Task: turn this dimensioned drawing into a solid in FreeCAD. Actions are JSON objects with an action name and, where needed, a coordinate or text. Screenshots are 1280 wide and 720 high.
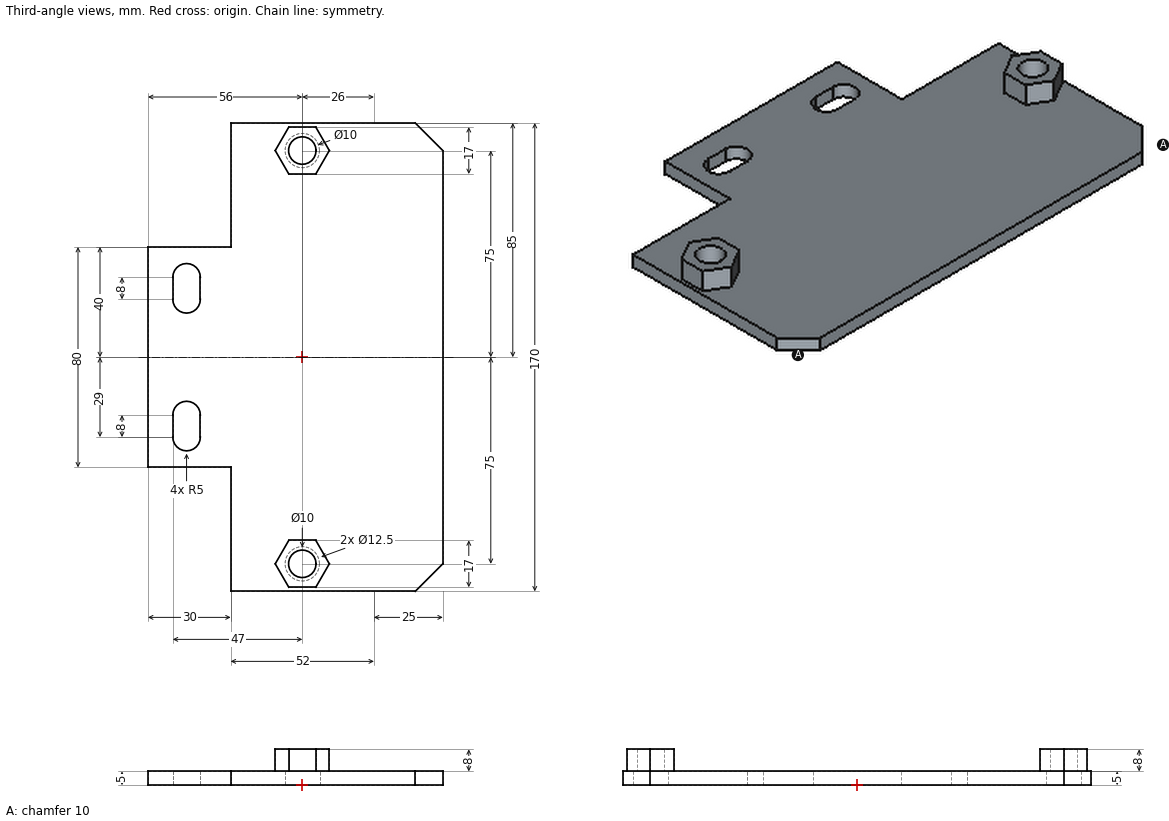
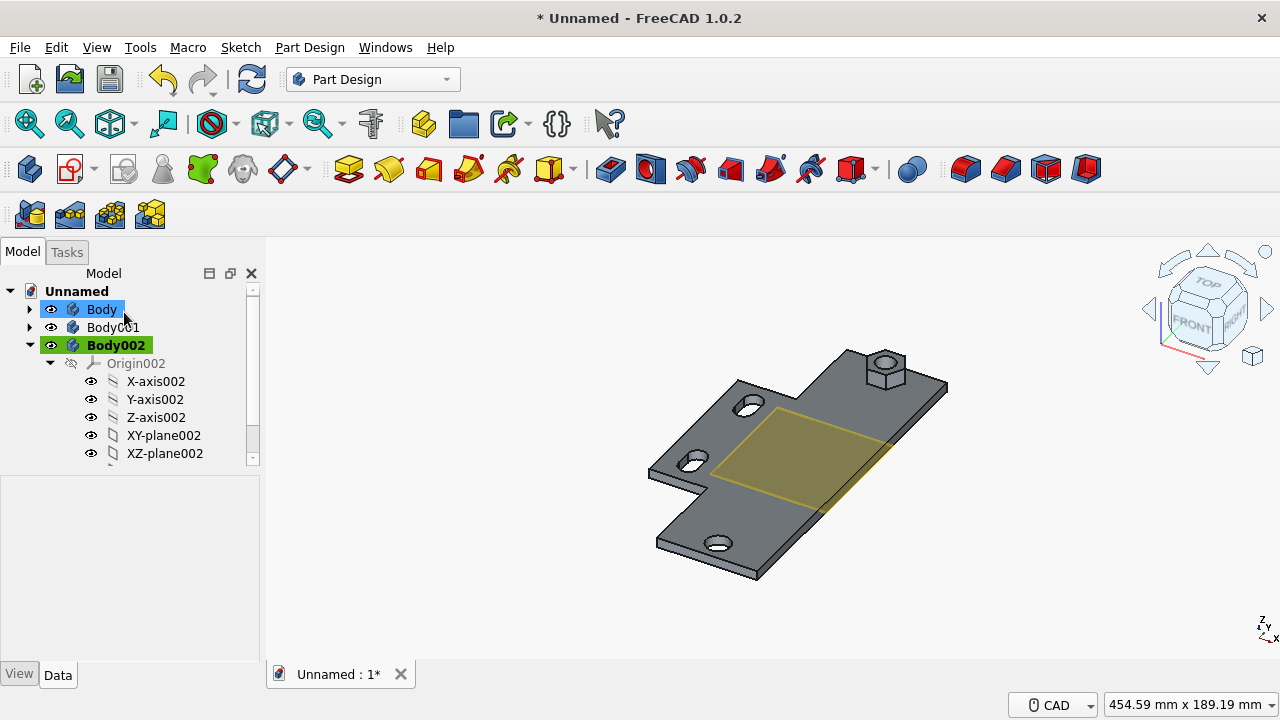
{"action": "scroll", "coordinate": [100, 377], "scroll_direction": "down", "scroll_amount": 3}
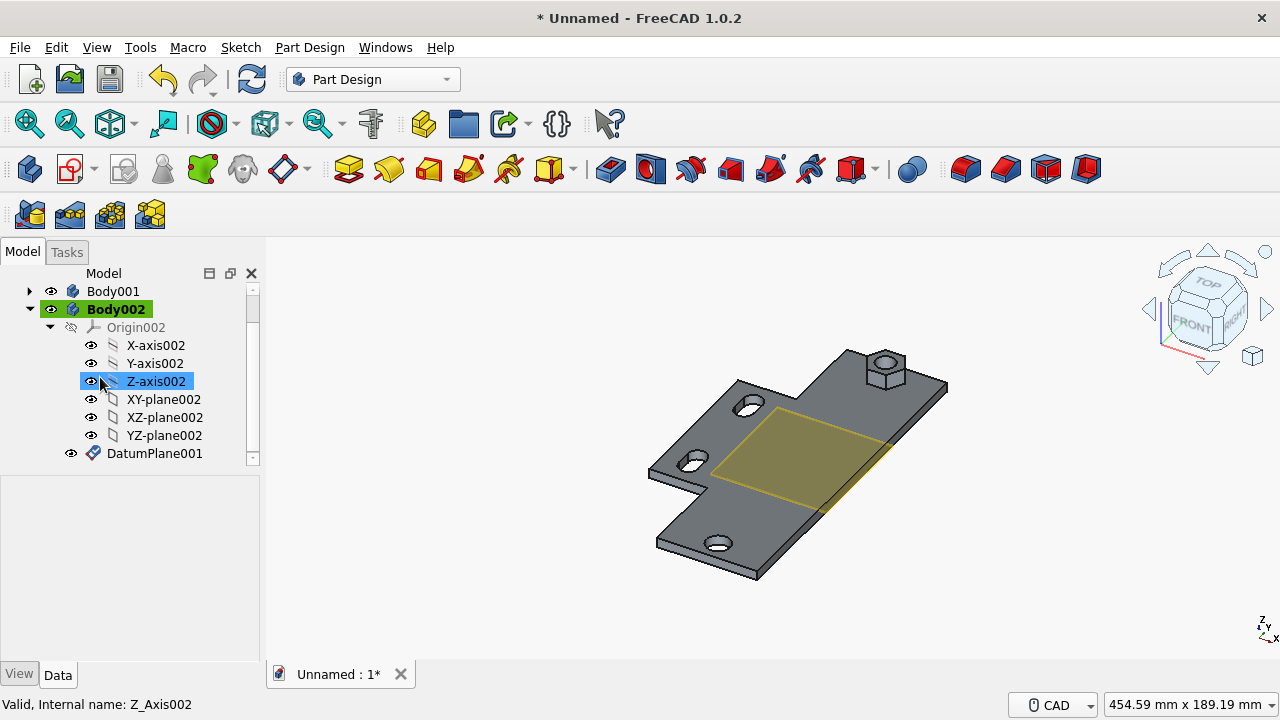
{"action": "left_click", "coordinate": [116, 453]}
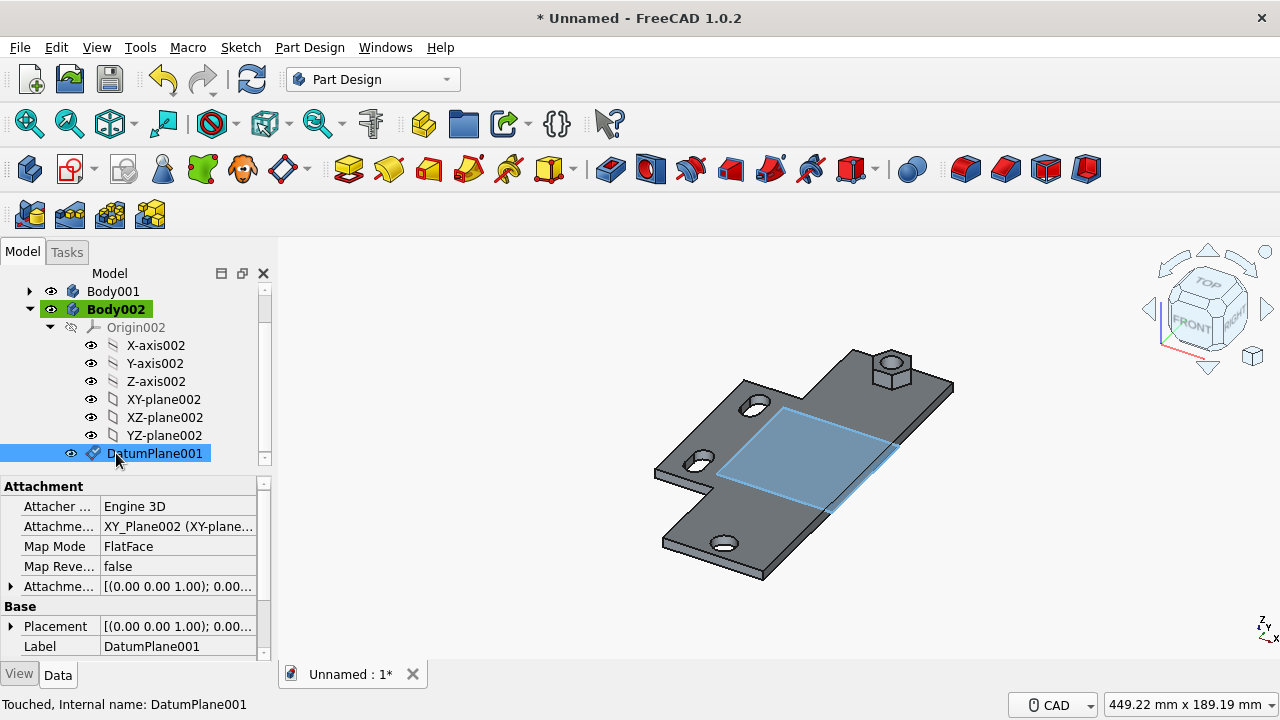
{"action": "left_click", "coordinate": [70, 170]}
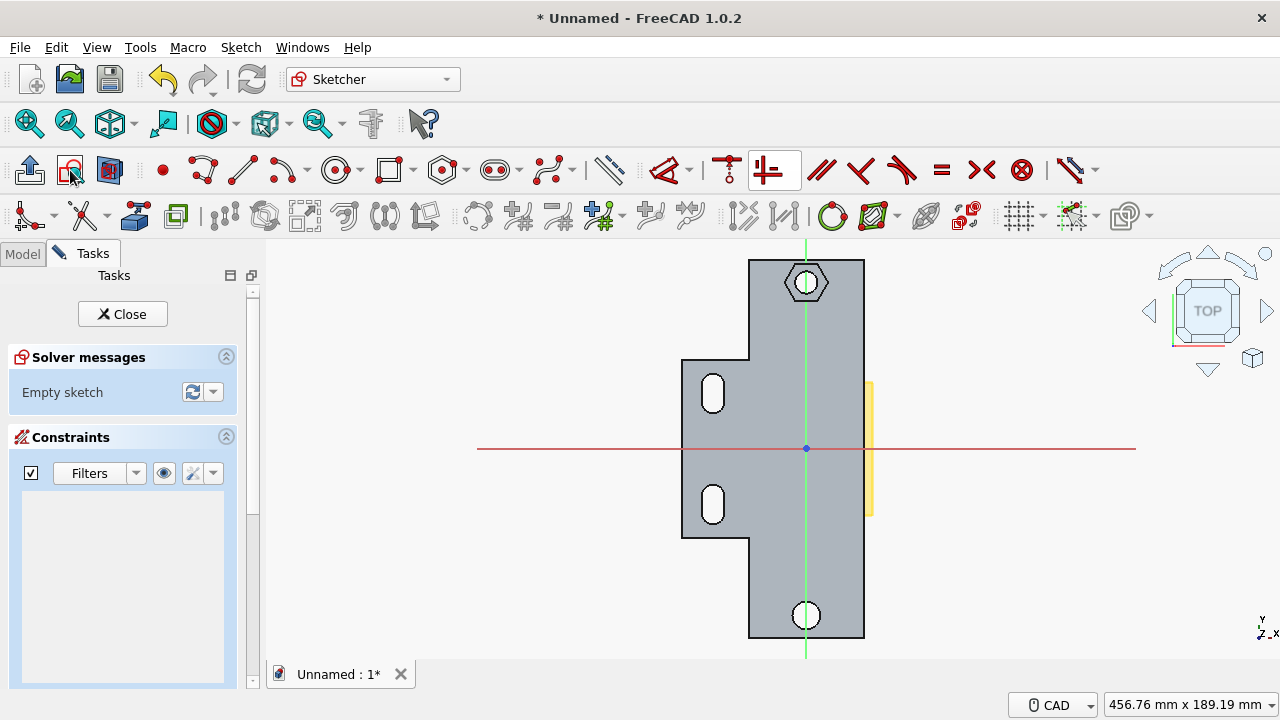
{"action": "scroll", "coordinate": [704, 449], "scroll_direction": "down", "scroll_amount": 5}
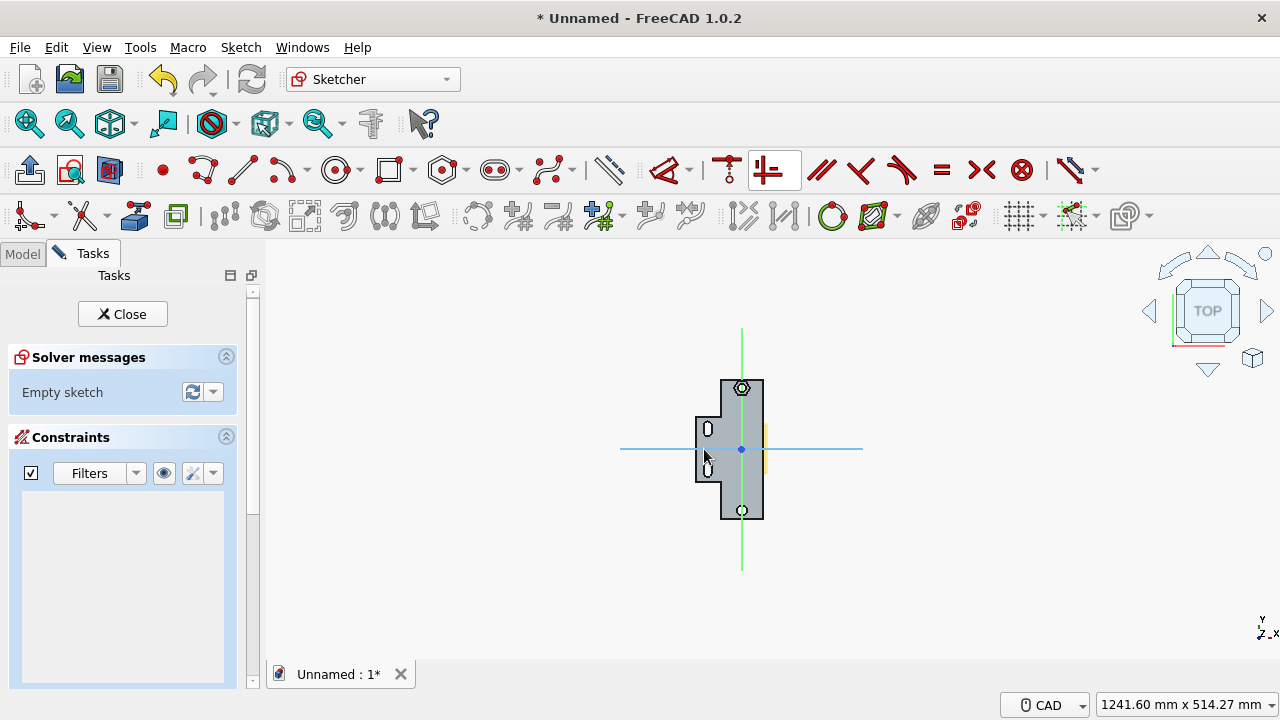
{"action": "scroll", "coordinate": [744, 514], "scroll_direction": "up", "scroll_amount": 15}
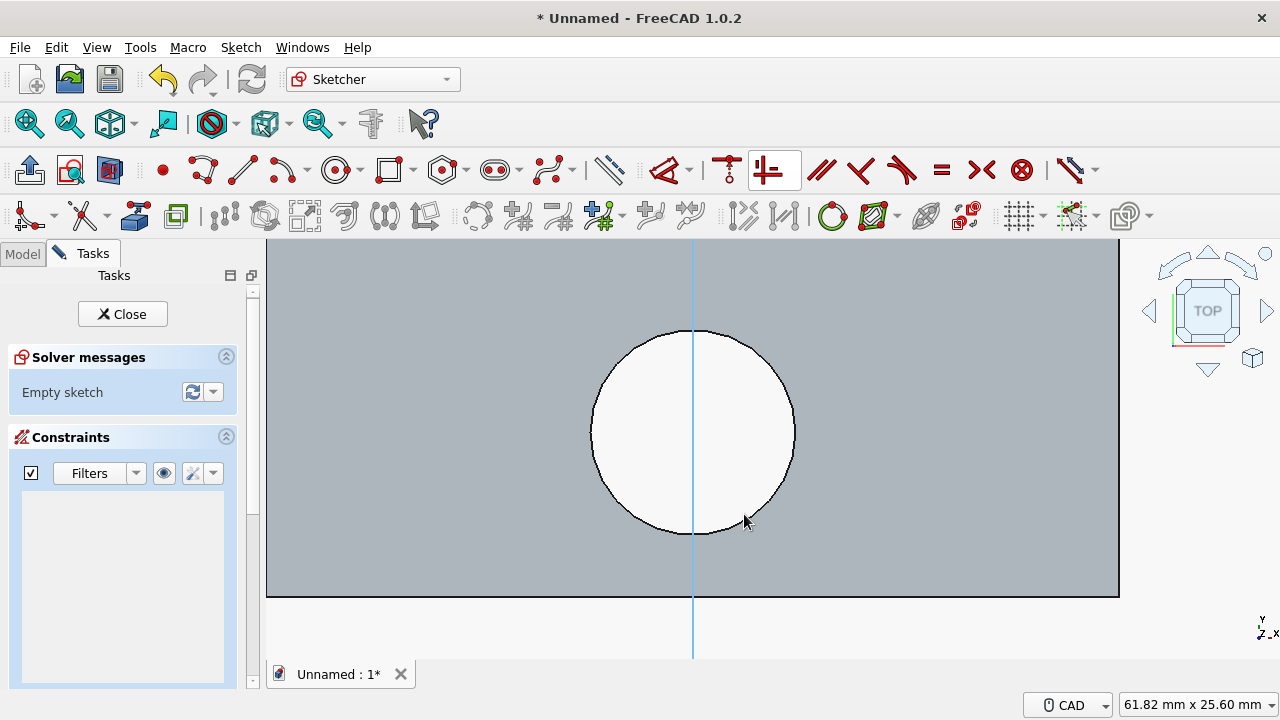
{"action": "left_click", "coordinate": [442, 170]}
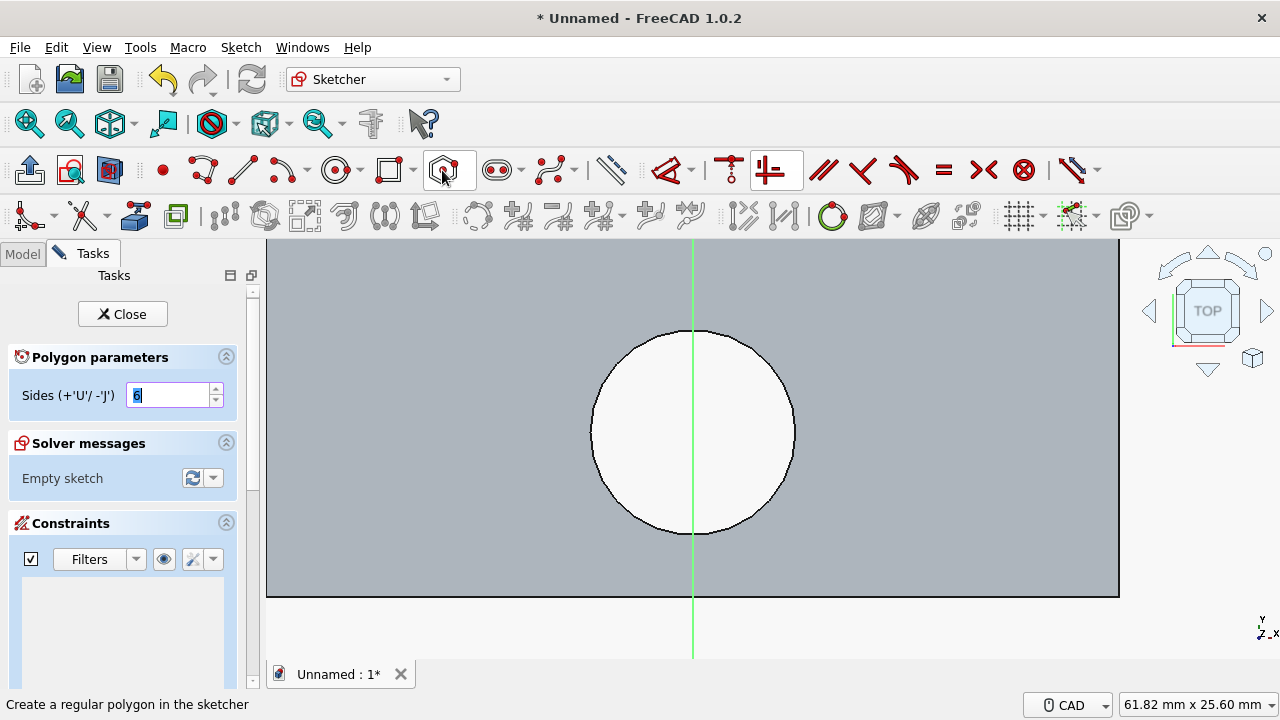
{"action": "left_click", "coordinate": [693, 433]}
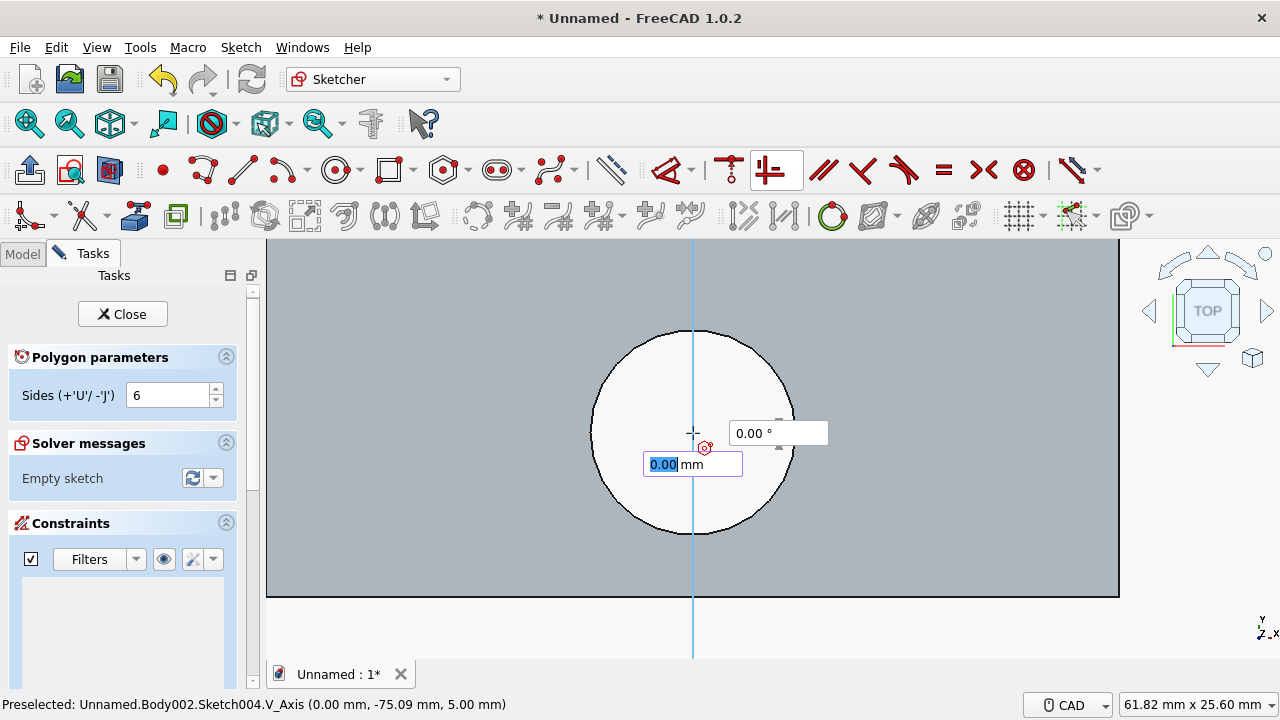
{"action": "left_click", "coordinate": [854, 433]}
{"action": "key", "text": "Escape"}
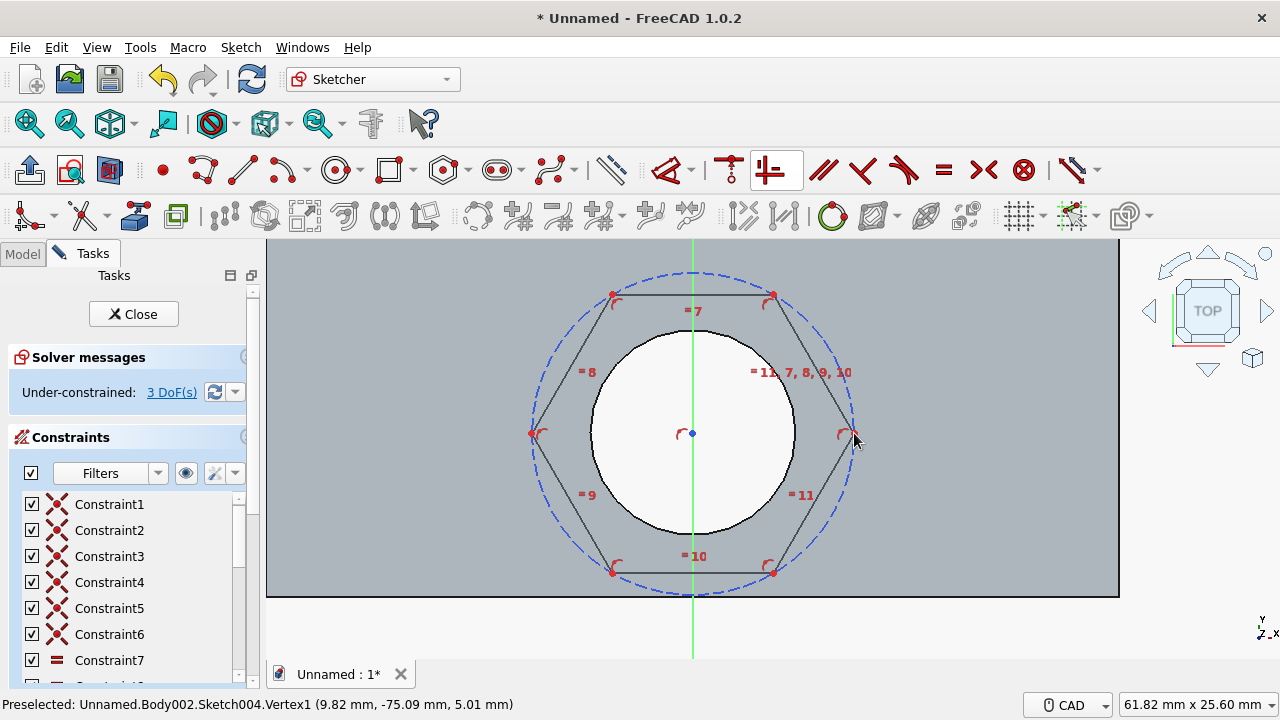
{"action": "left_click", "coordinate": [336, 170]}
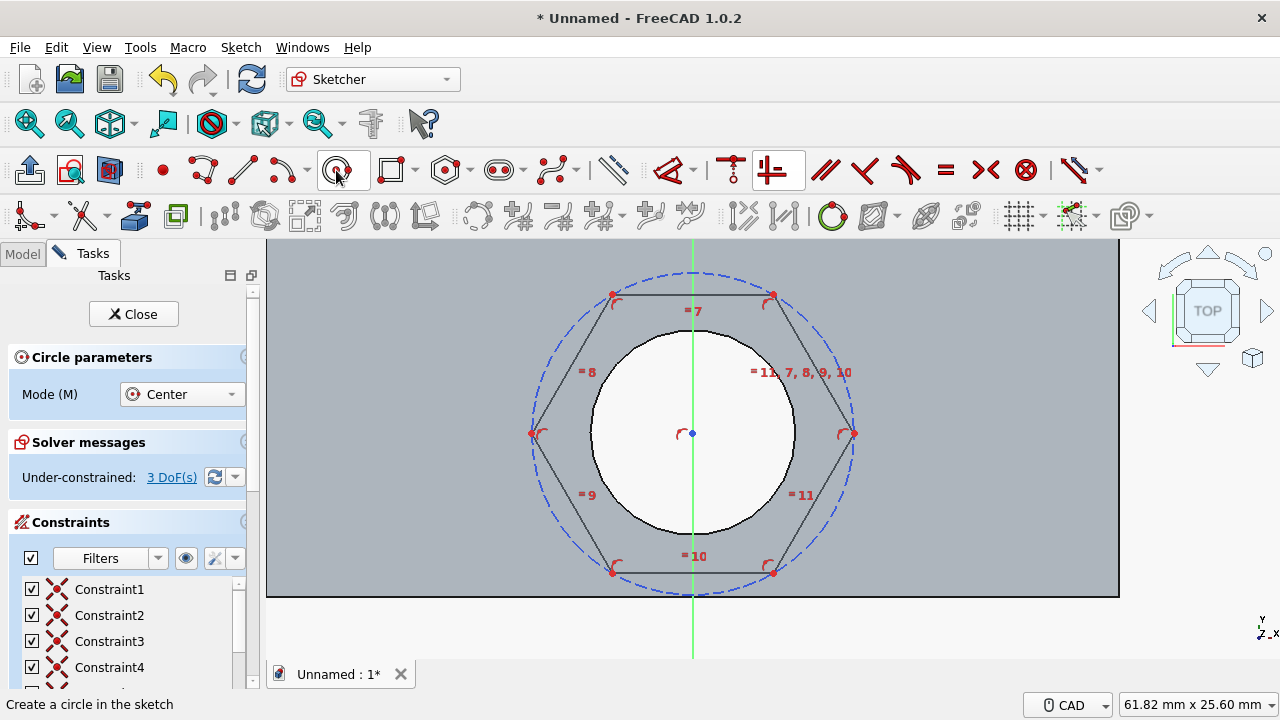
{"action": "left_click", "coordinate": [693, 434]}
{"action": "left_click", "coordinate": [751, 375]}
{"action": "key", "text": "Escape"}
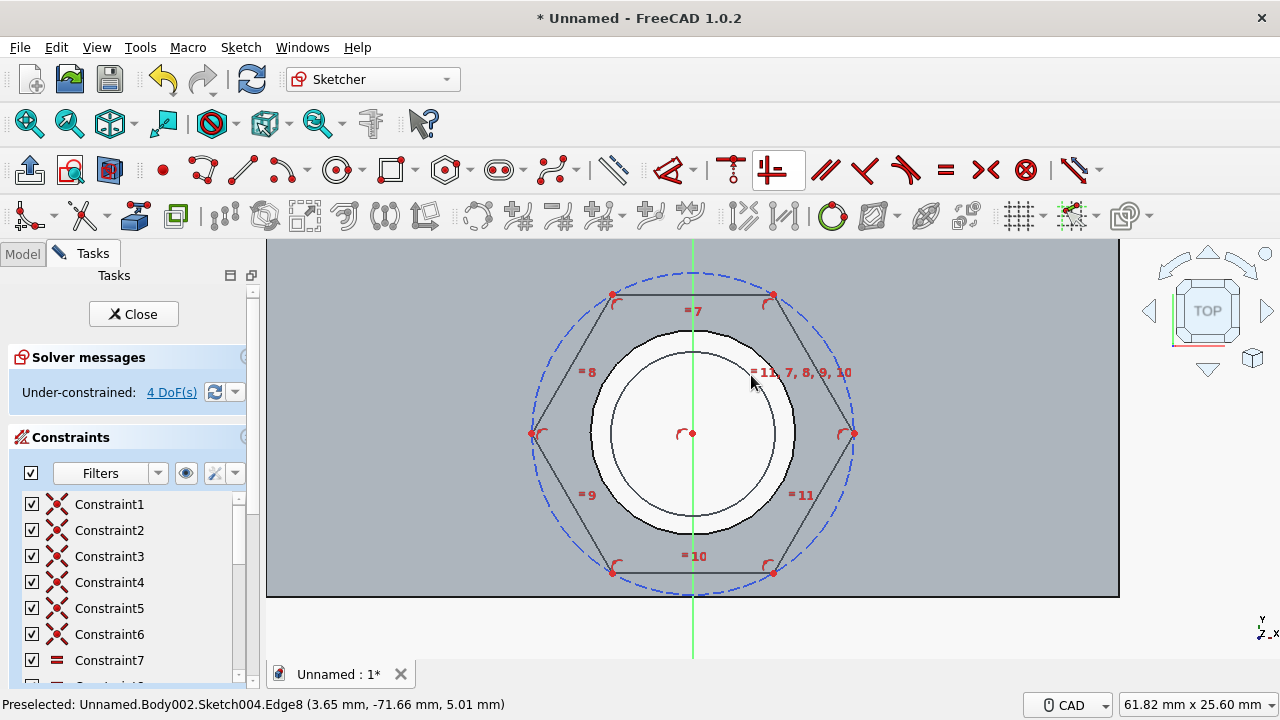
{"action": "left_click", "coordinate": [725, 295]}